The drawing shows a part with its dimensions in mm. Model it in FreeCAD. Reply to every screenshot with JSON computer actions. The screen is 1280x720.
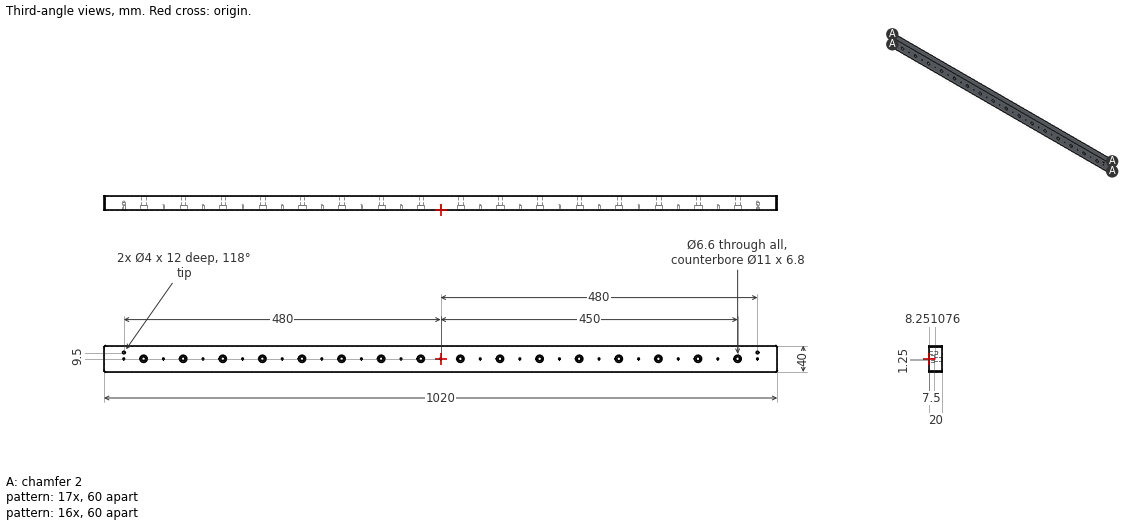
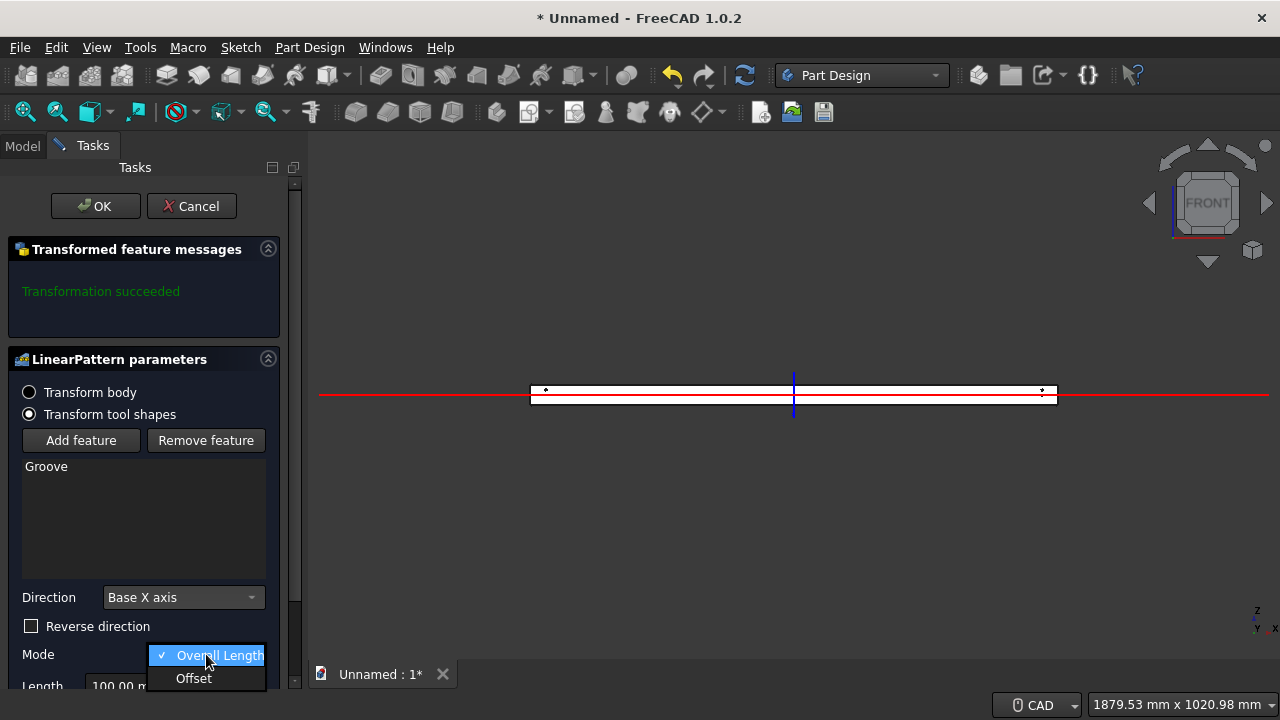
{"action": "left_click", "coordinate": [206, 678]}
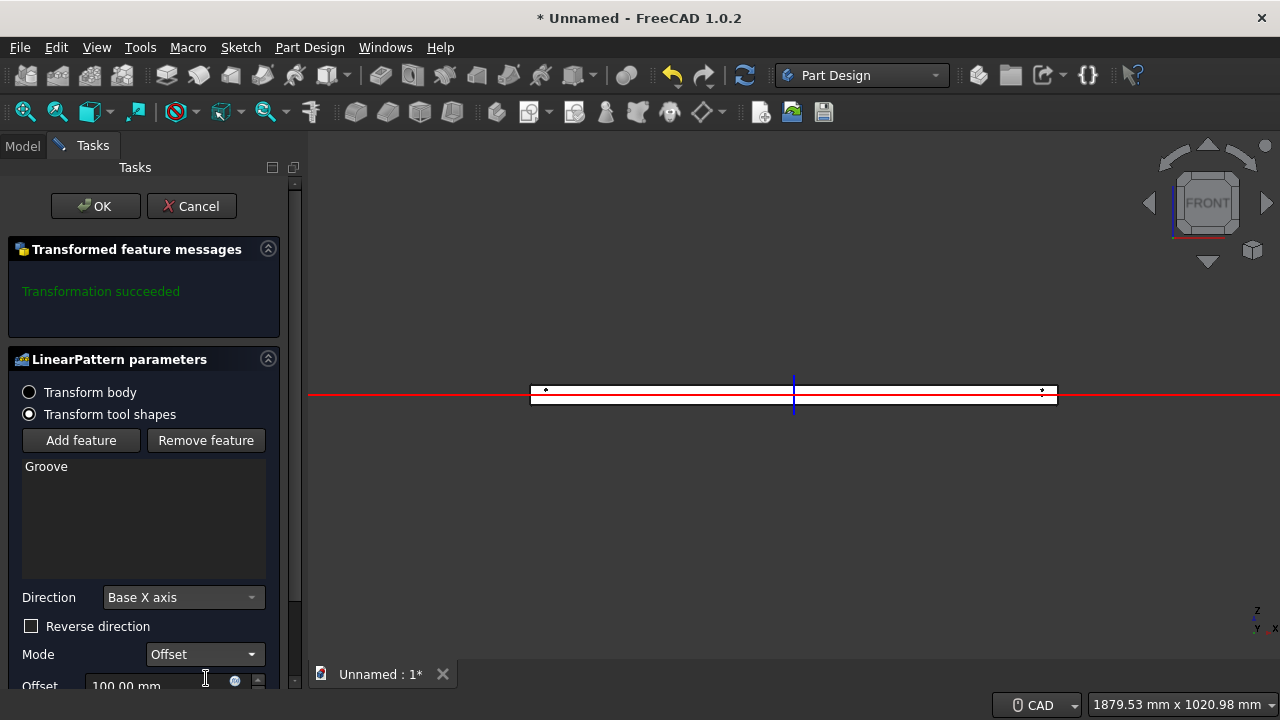
{"action": "scroll", "coordinate": [295, 432], "scroll_direction": "down", "scroll_amount": 2}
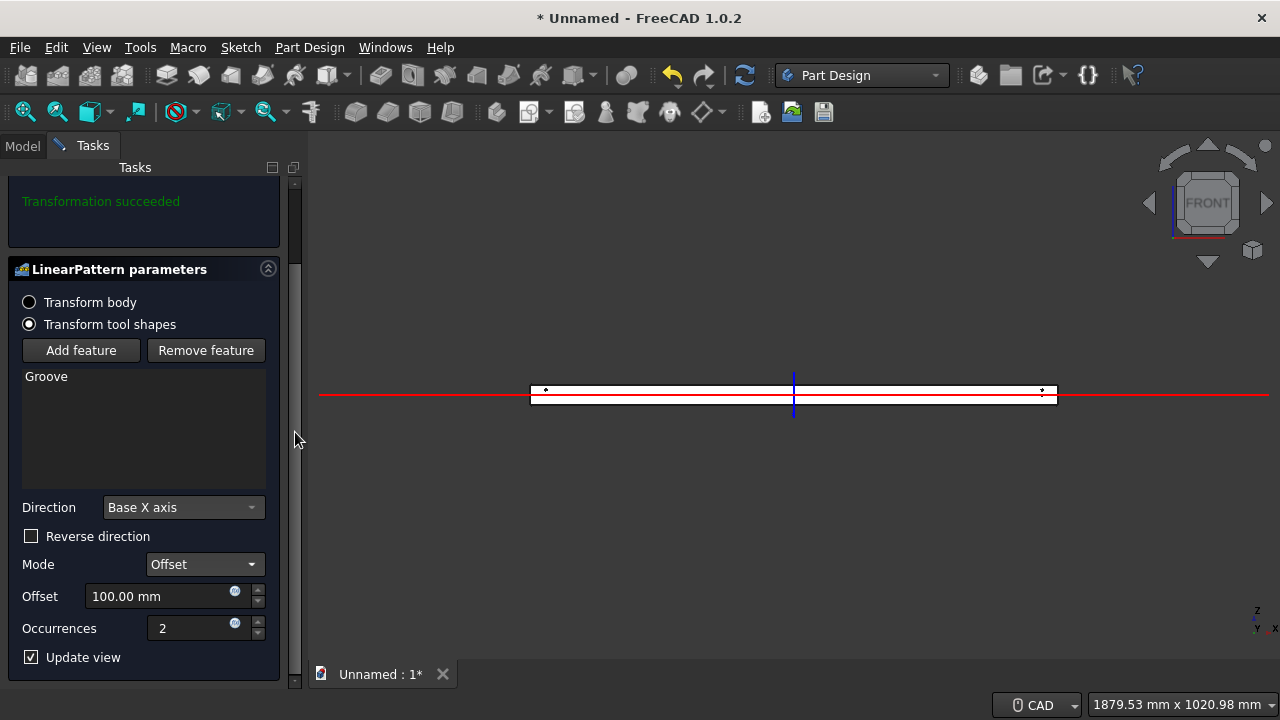
{"action": "triple_click", "coordinate": [168, 596]}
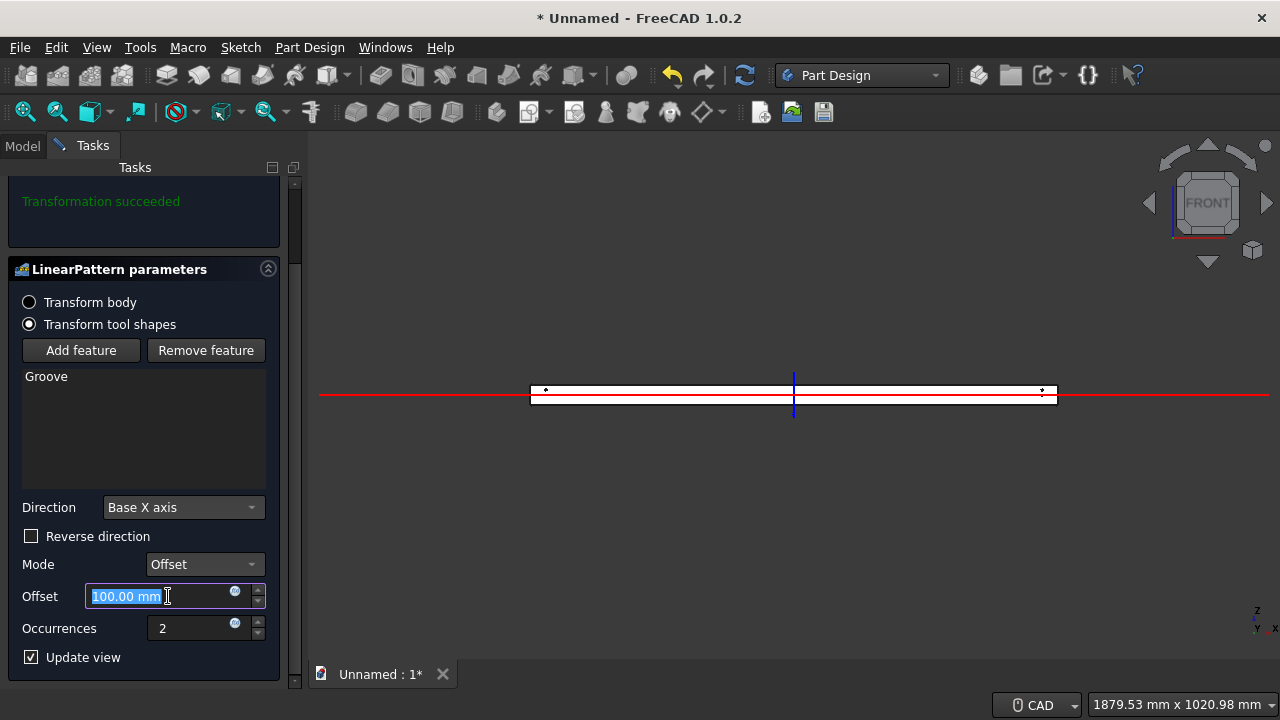
{"action": "type", "text": "60"}
{"action": "key", "text": "Tab"}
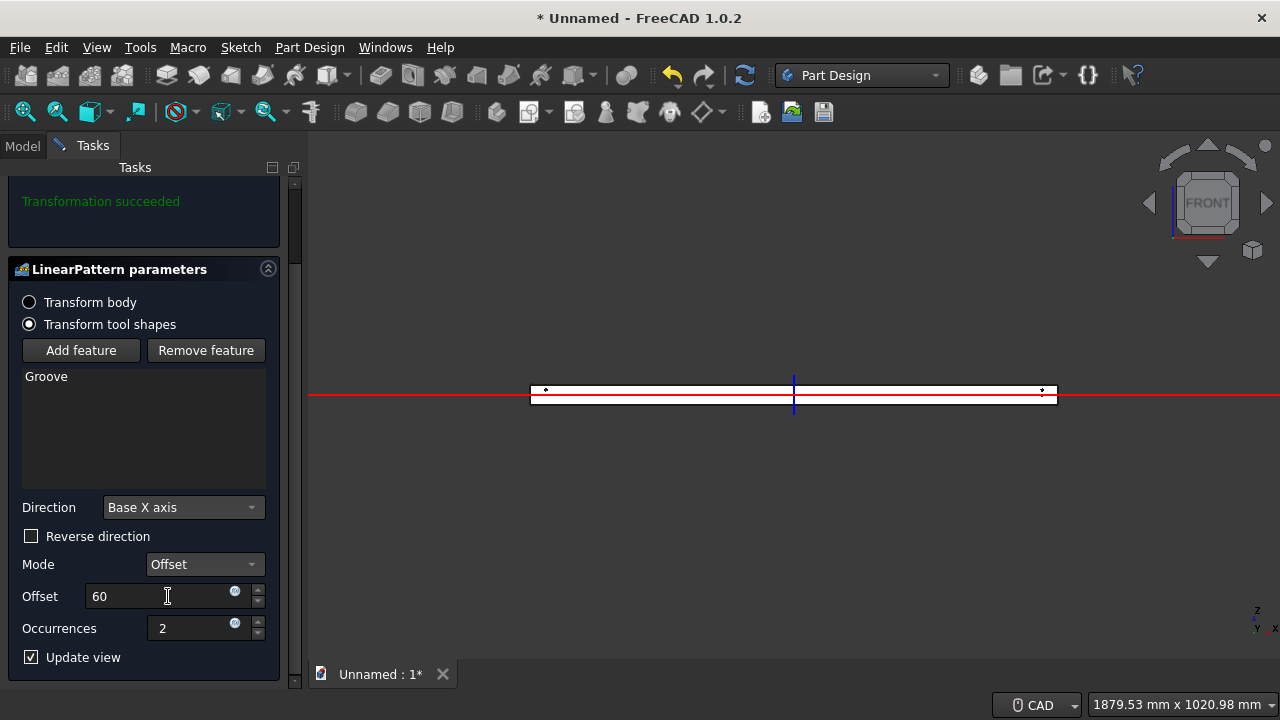
{"action": "triple_click", "coordinate": [198, 628]}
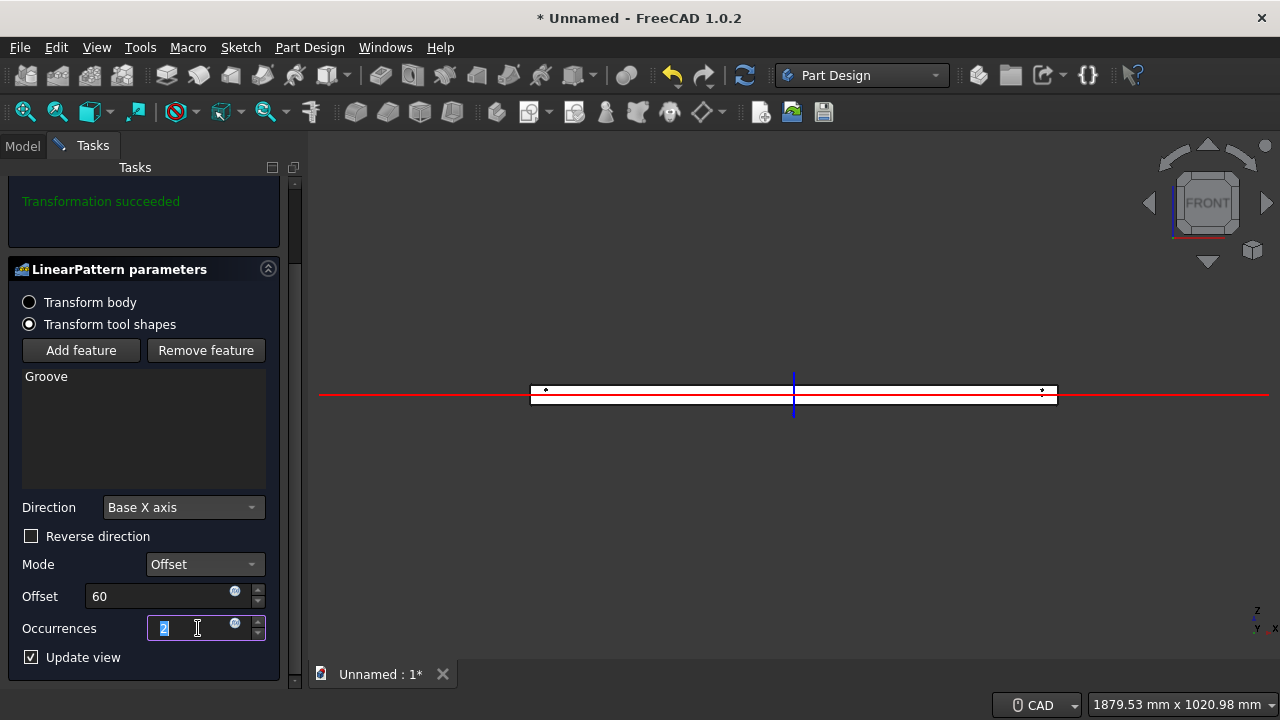
{"action": "type", "text": "17"}
{"action": "key", "text": "Tab"}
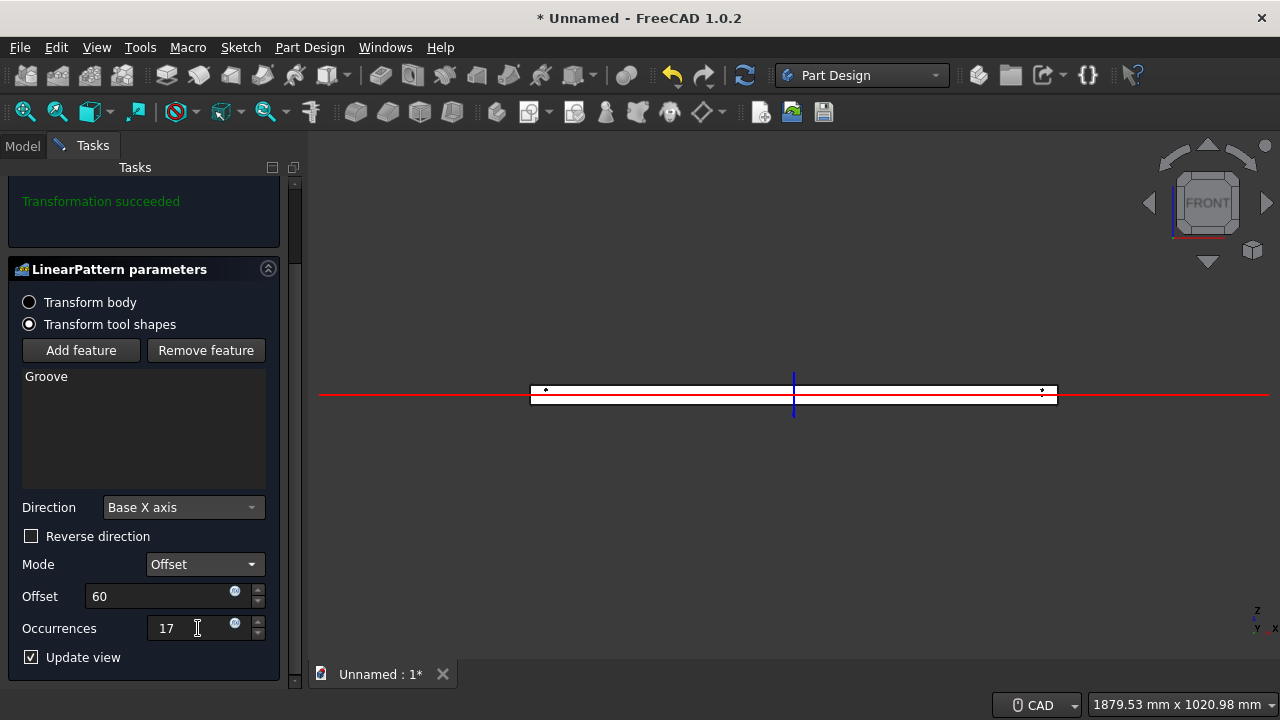
{"action": "left_click", "coordinate": [30, 536]}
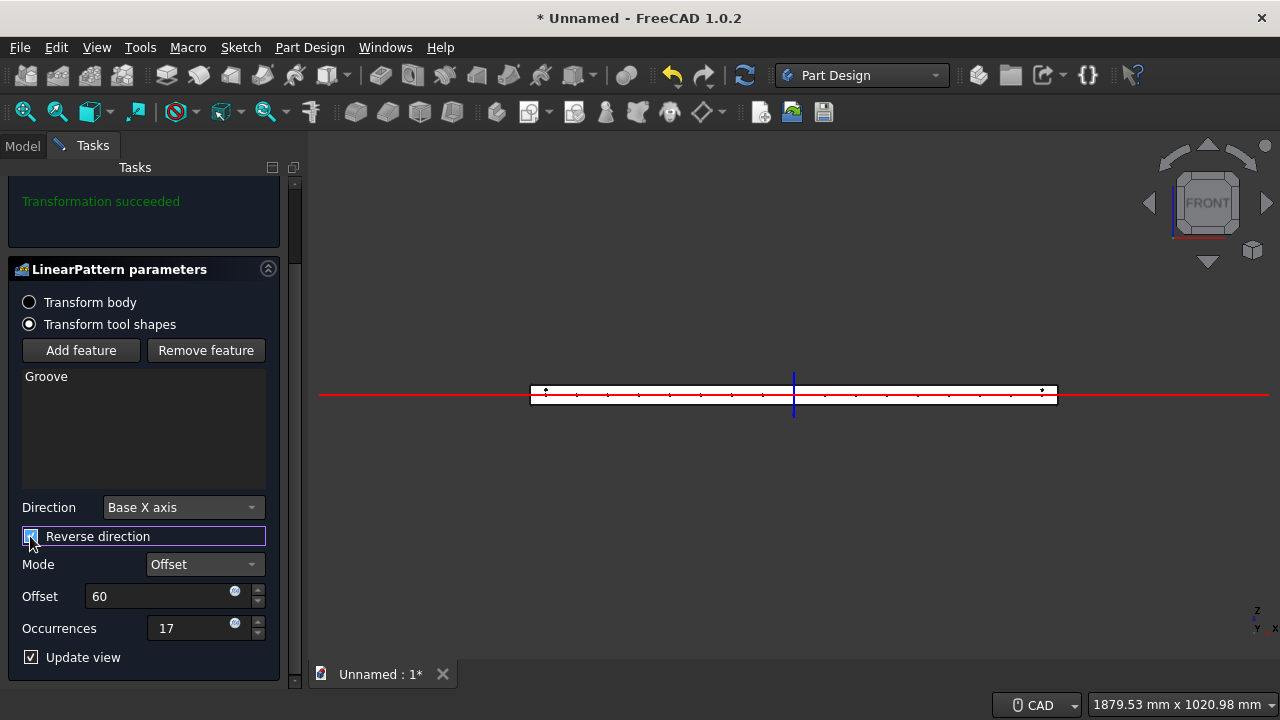
{"action": "scroll", "coordinate": [295, 432], "scroll_direction": "up", "scroll_amount": 3}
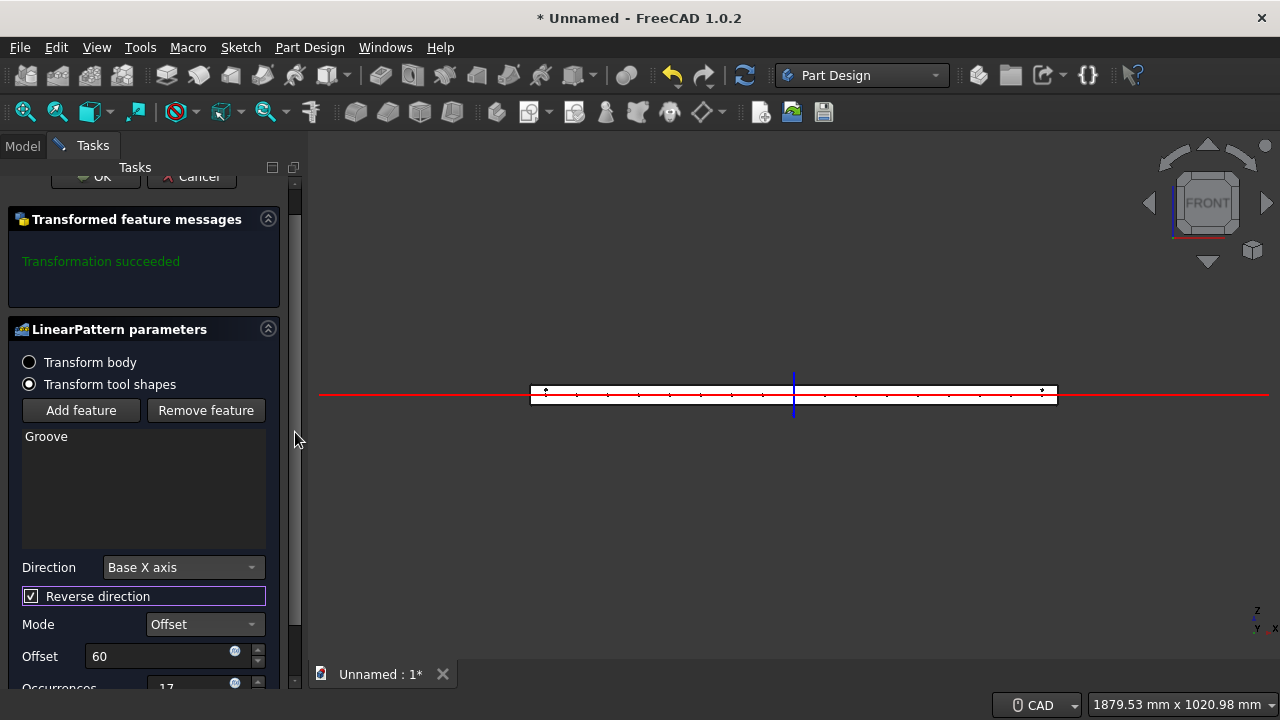
{"action": "left_click", "coordinate": [96, 206]}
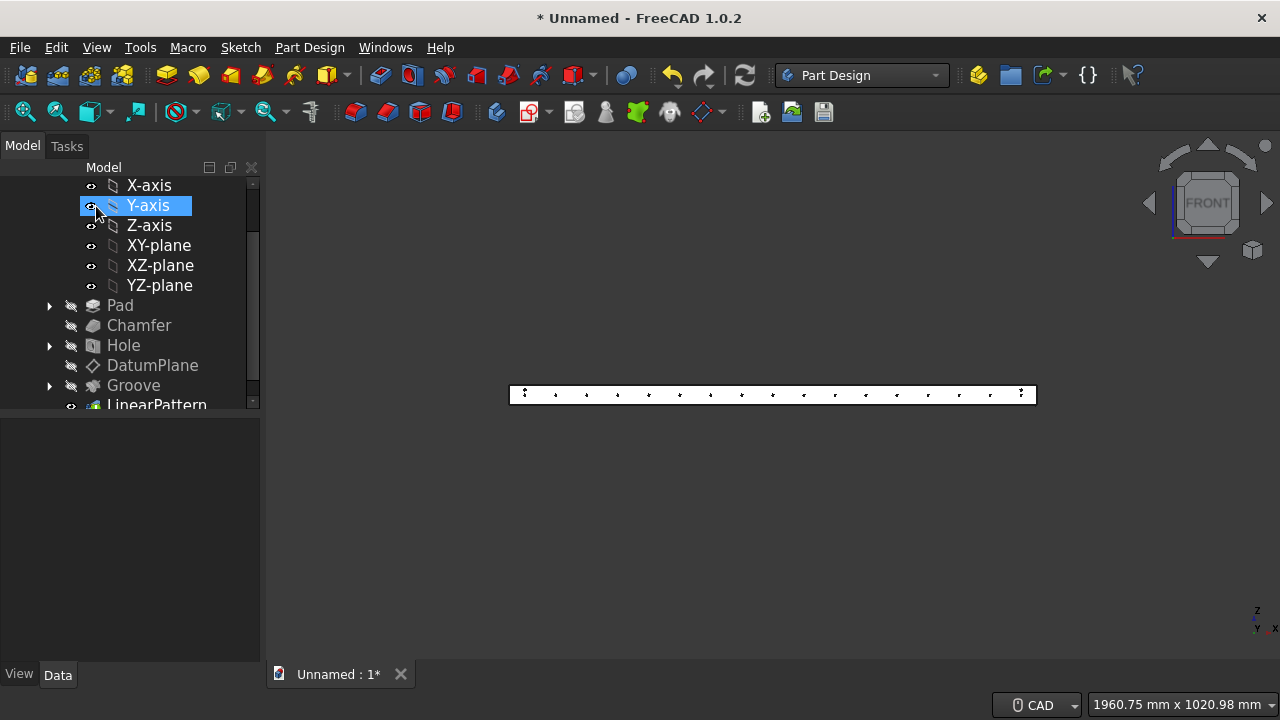
{"action": "left_click", "coordinate": [848, 394]}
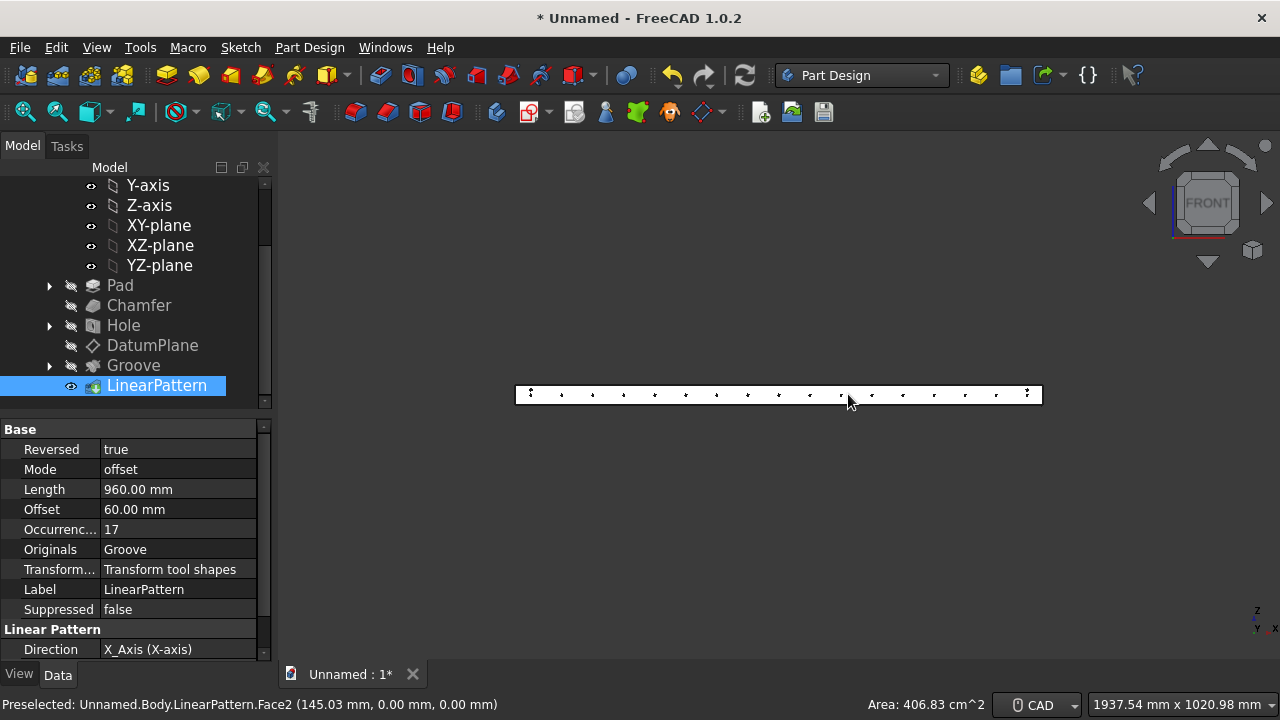
{"action": "left_click", "coordinate": [530, 112]}